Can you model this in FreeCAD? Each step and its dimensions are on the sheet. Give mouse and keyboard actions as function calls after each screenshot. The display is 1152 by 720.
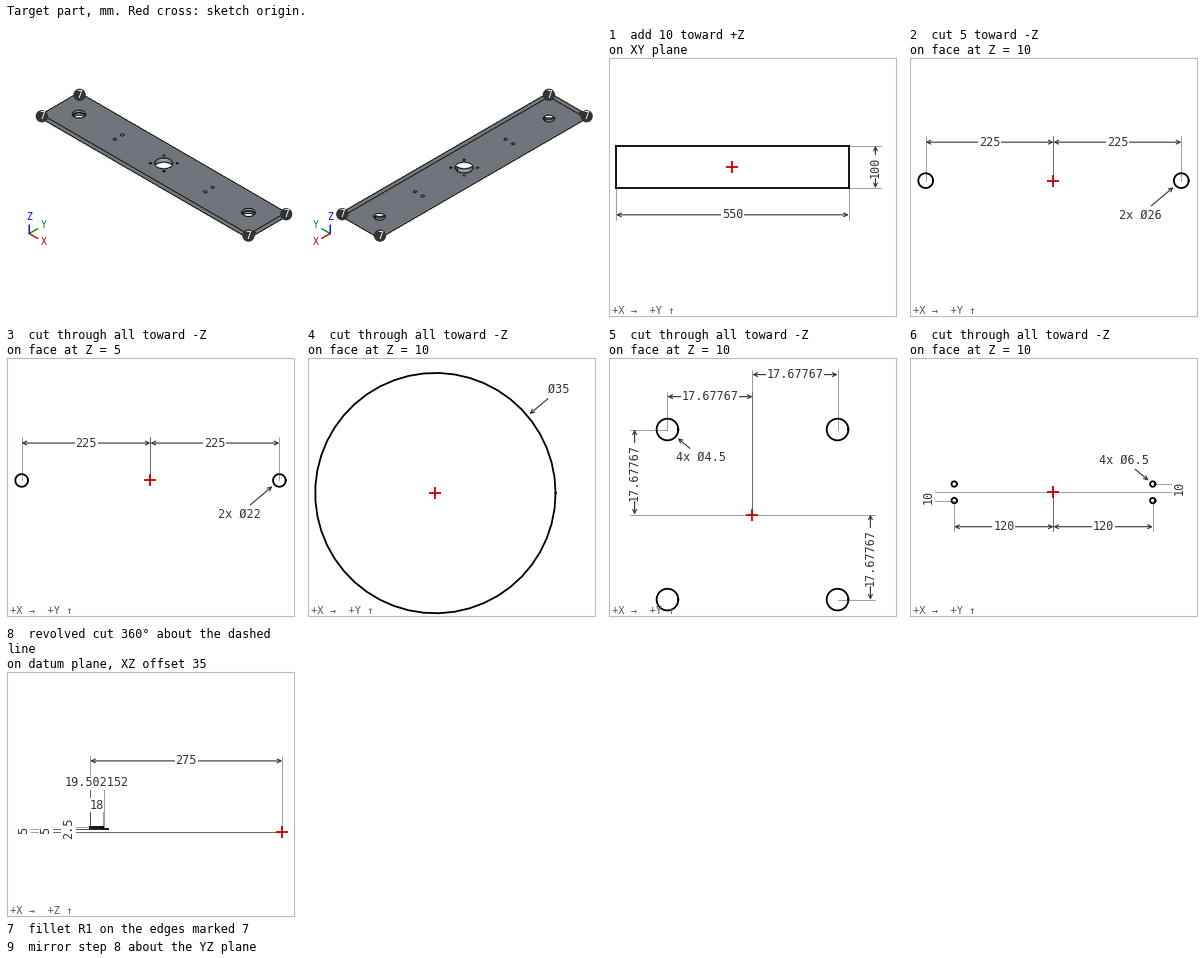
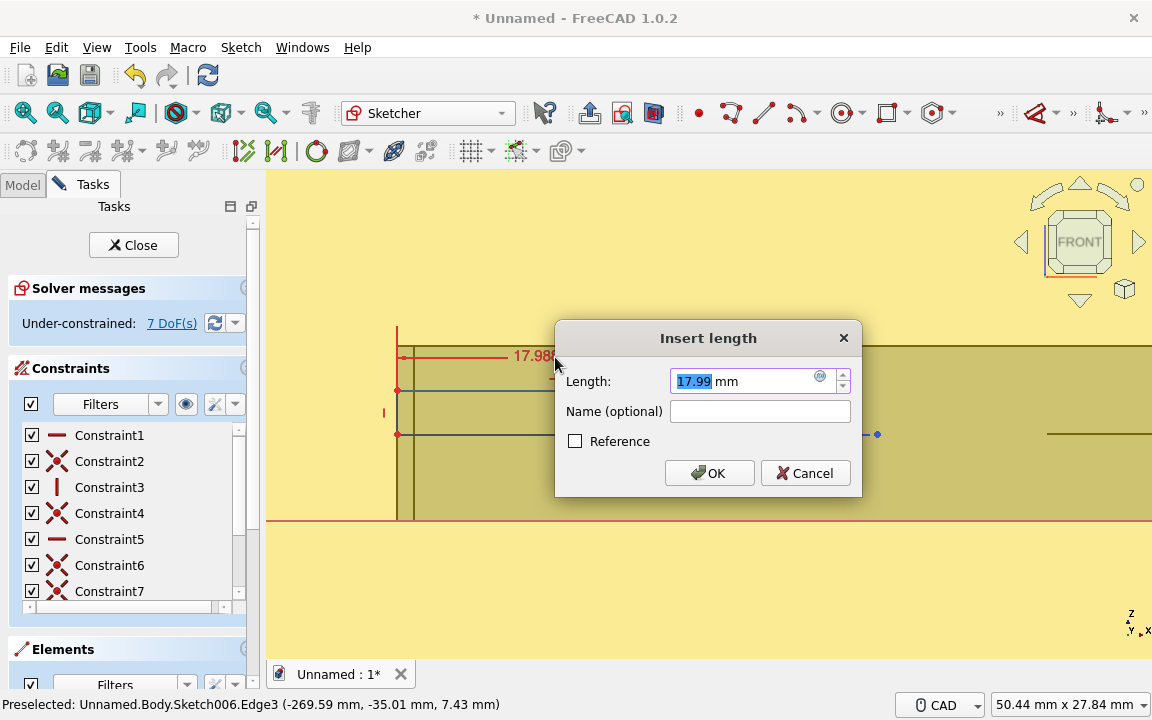
text(18)
key(Return)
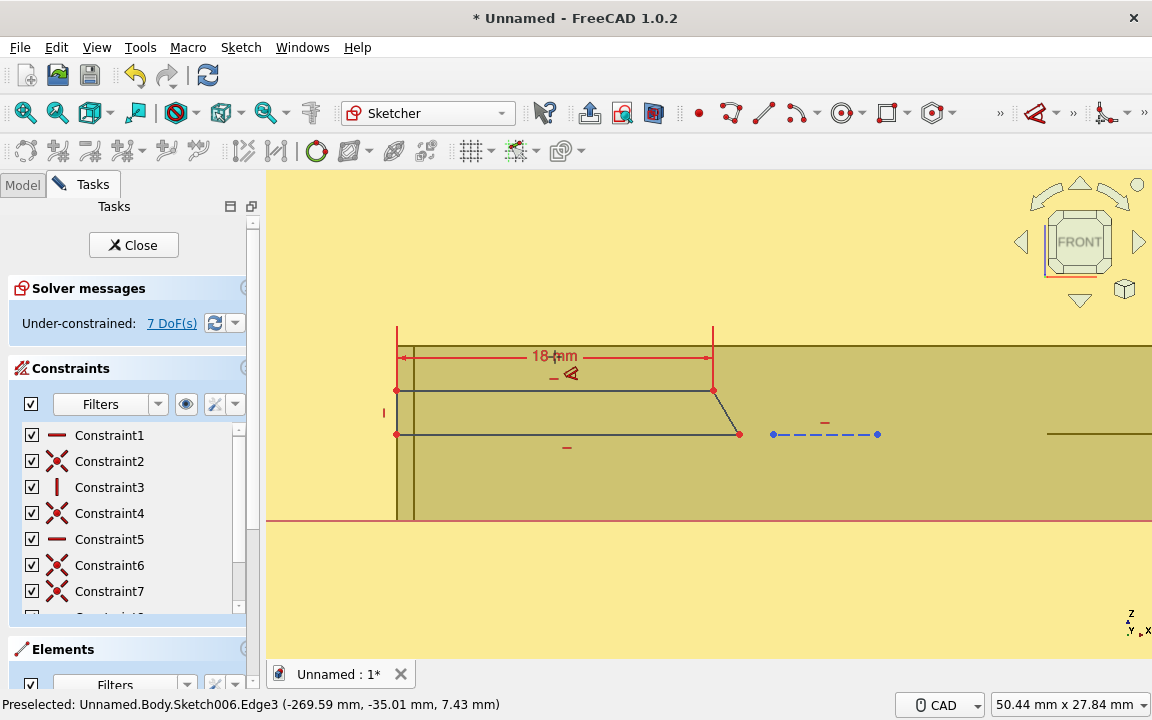
click(739, 435)
click(705, 478)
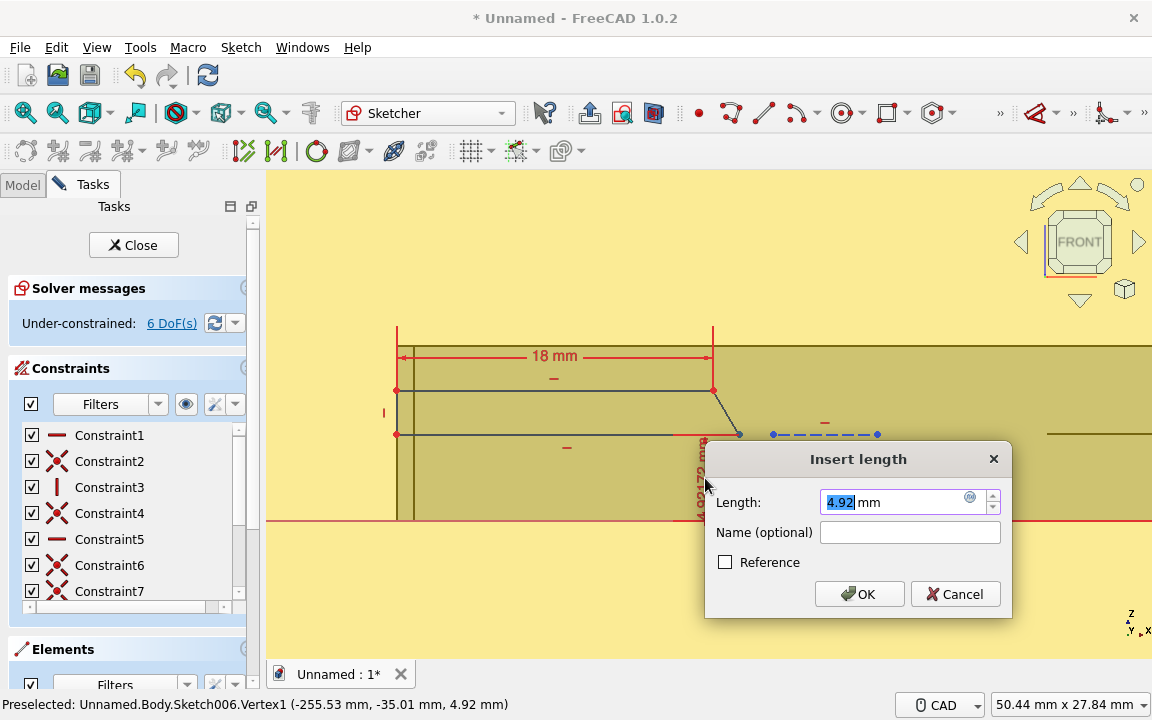
text(5)
key(Return)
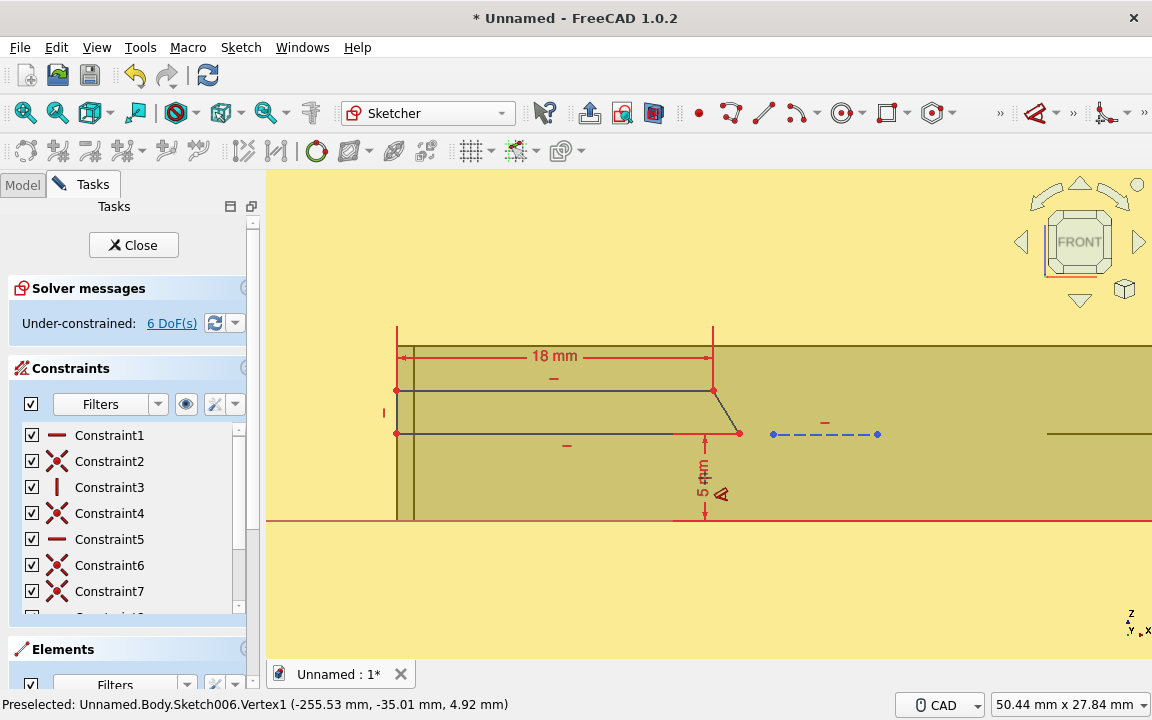
click(774, 435)
click(740, 448)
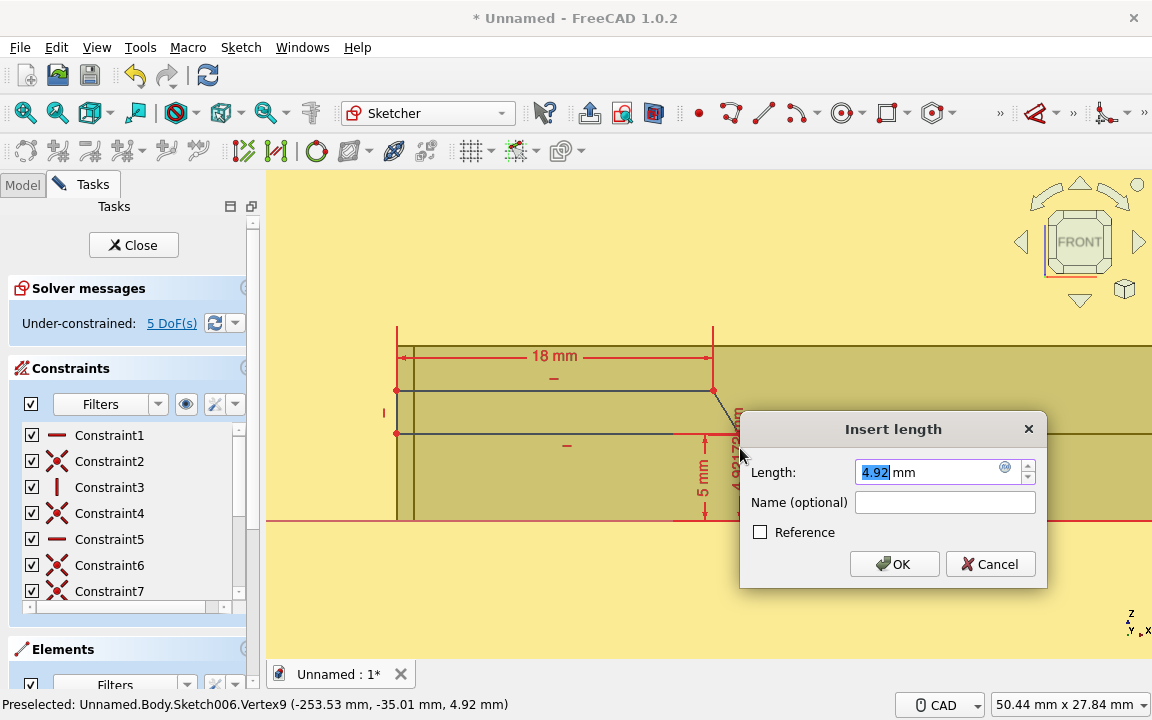
text(5)
key(Return)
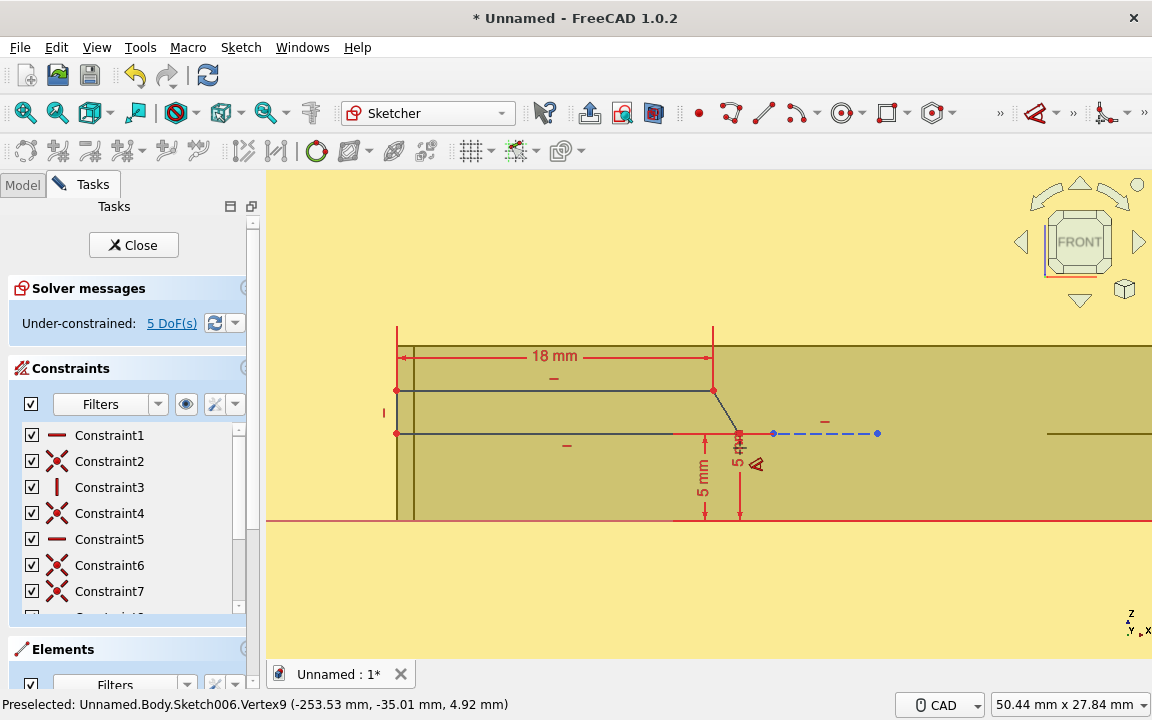
click(397, 421)
click(363, 412)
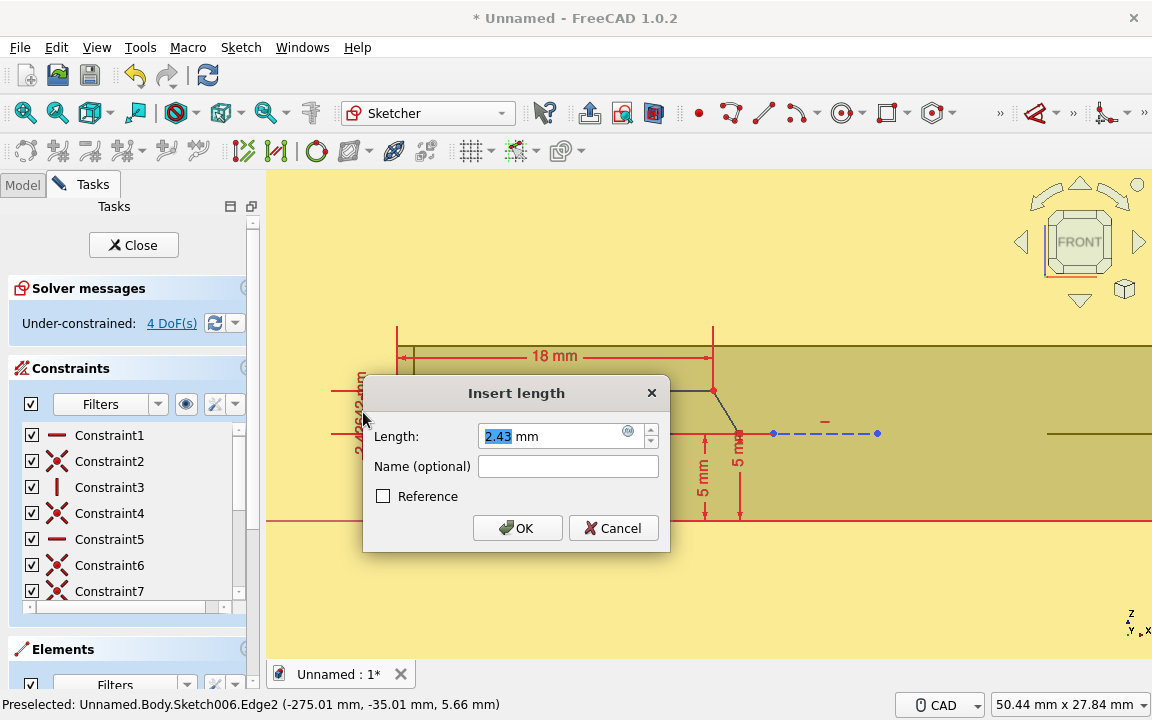
text(2.5)
key(Return)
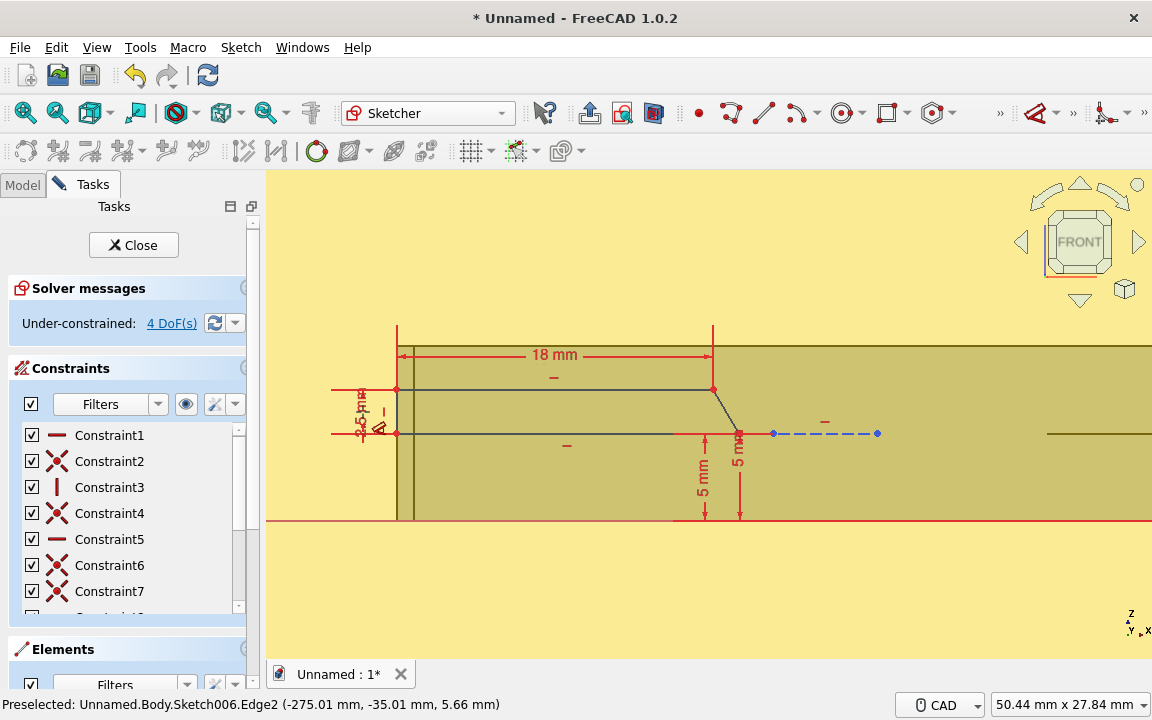
click(397, 434)
click(692, 555)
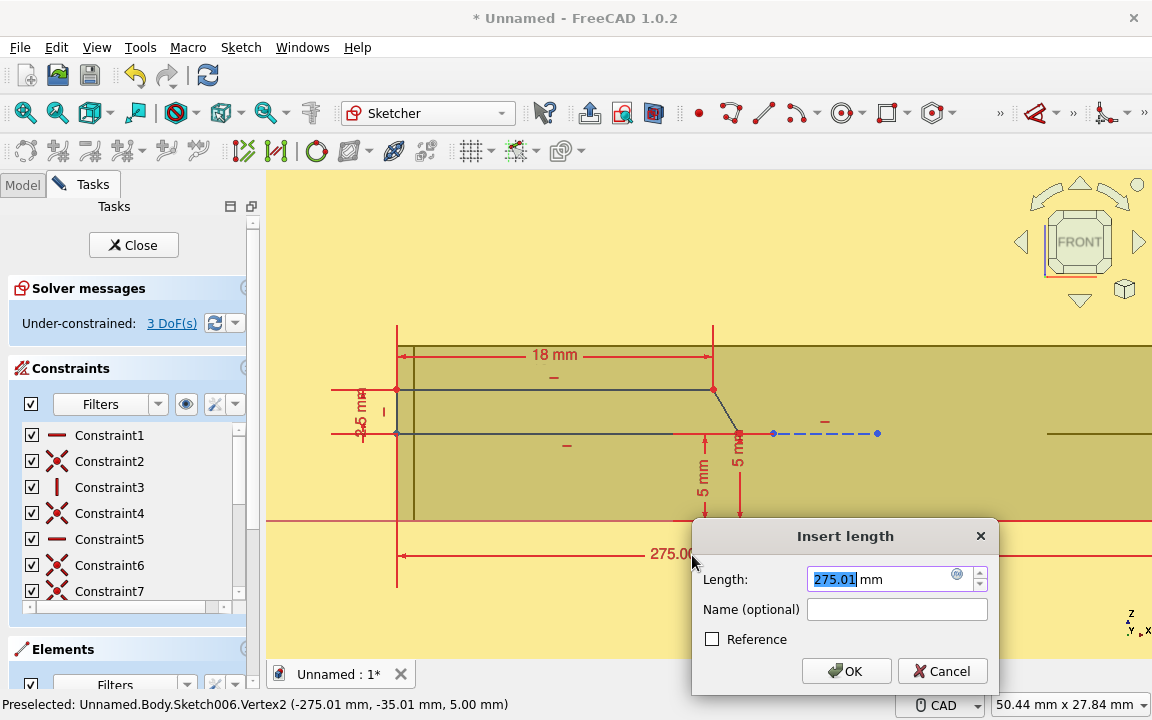
text(275)
key(Return)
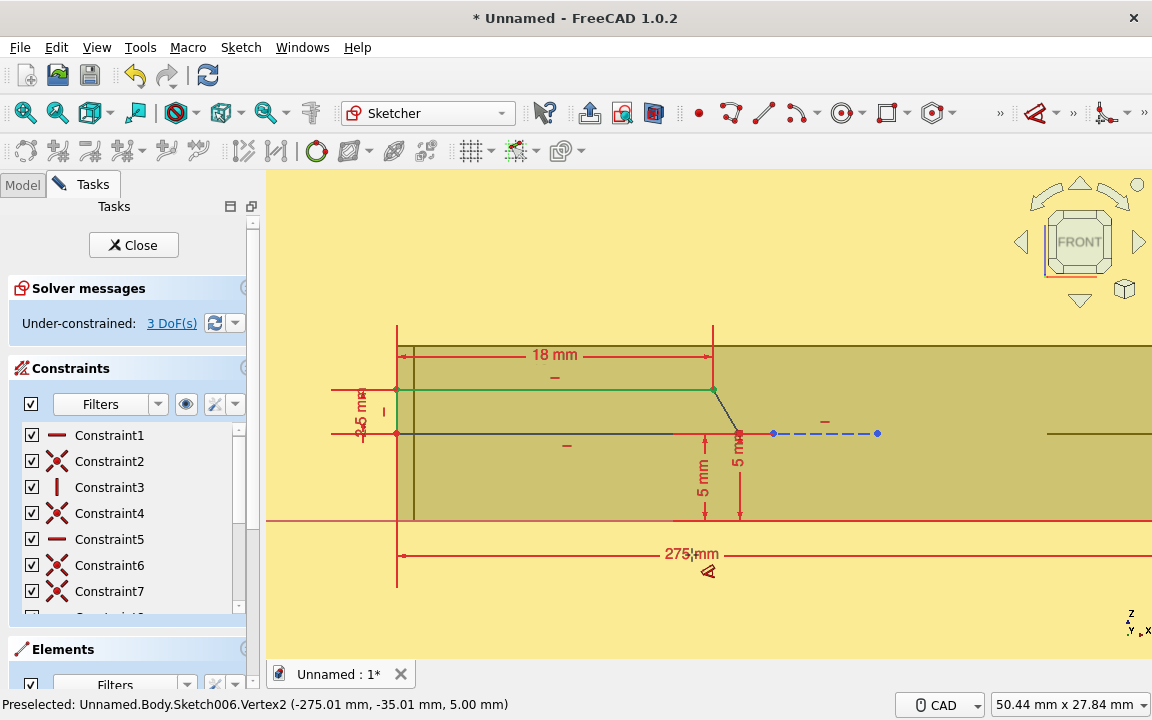
click(636, 434)
click(568, 468)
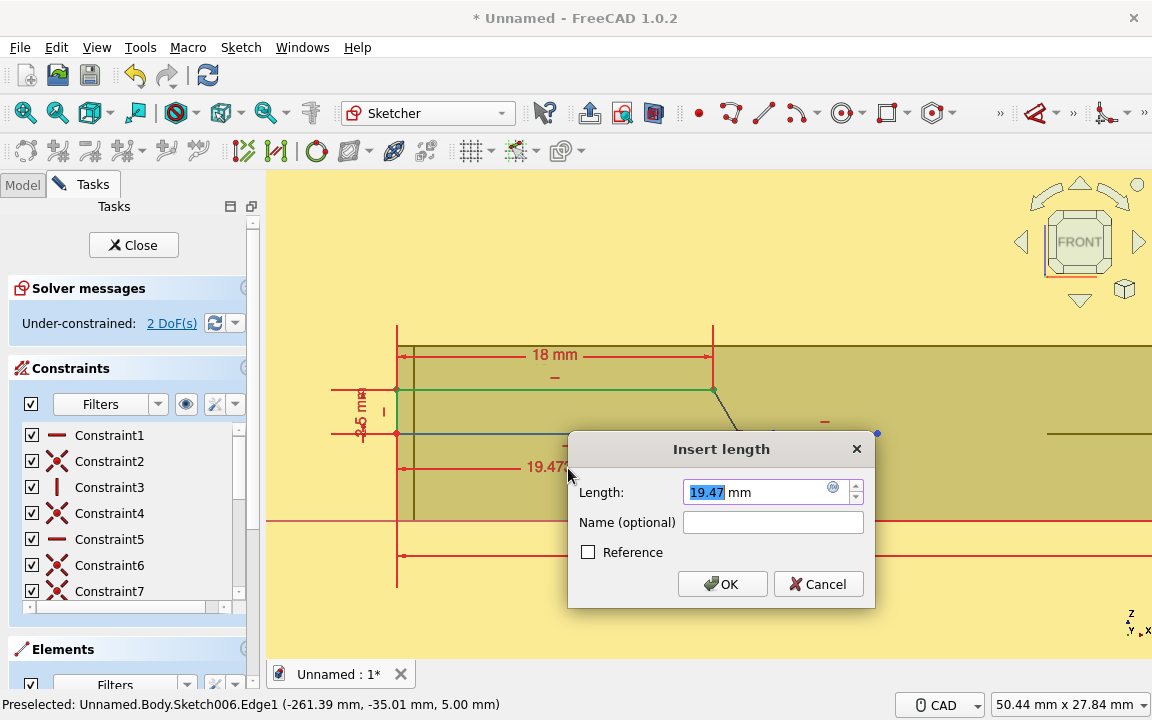
text(19.502152)
key(Return)
key(Escape)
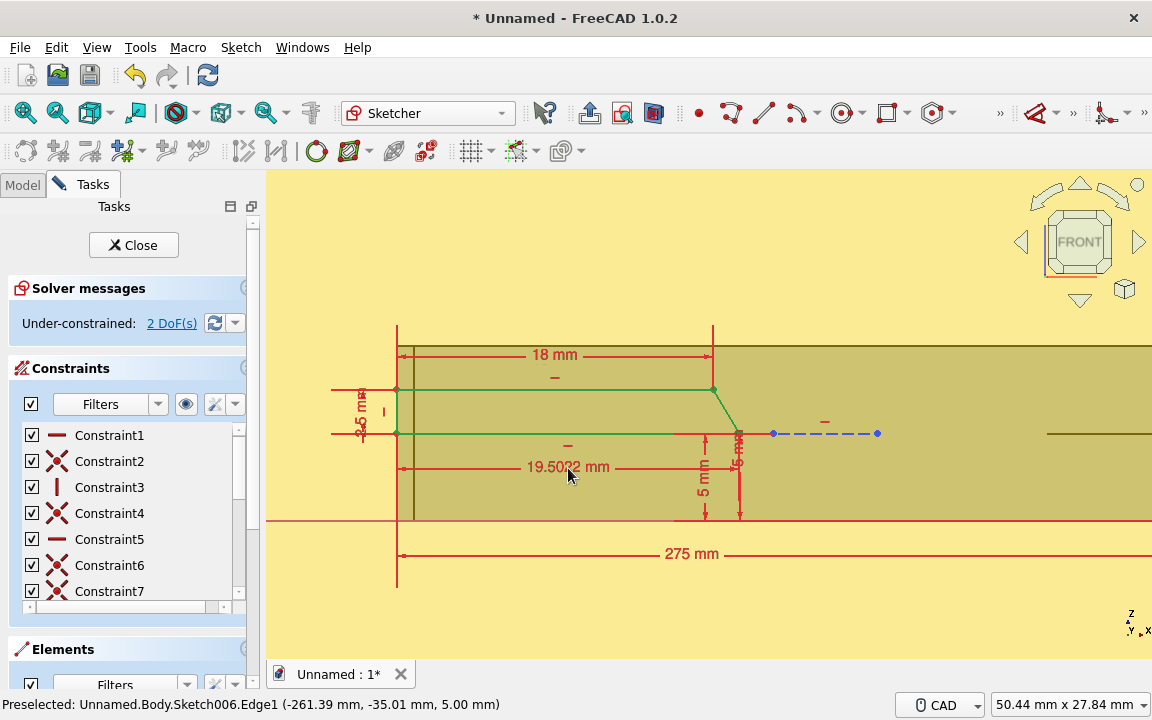
click(134, 245)